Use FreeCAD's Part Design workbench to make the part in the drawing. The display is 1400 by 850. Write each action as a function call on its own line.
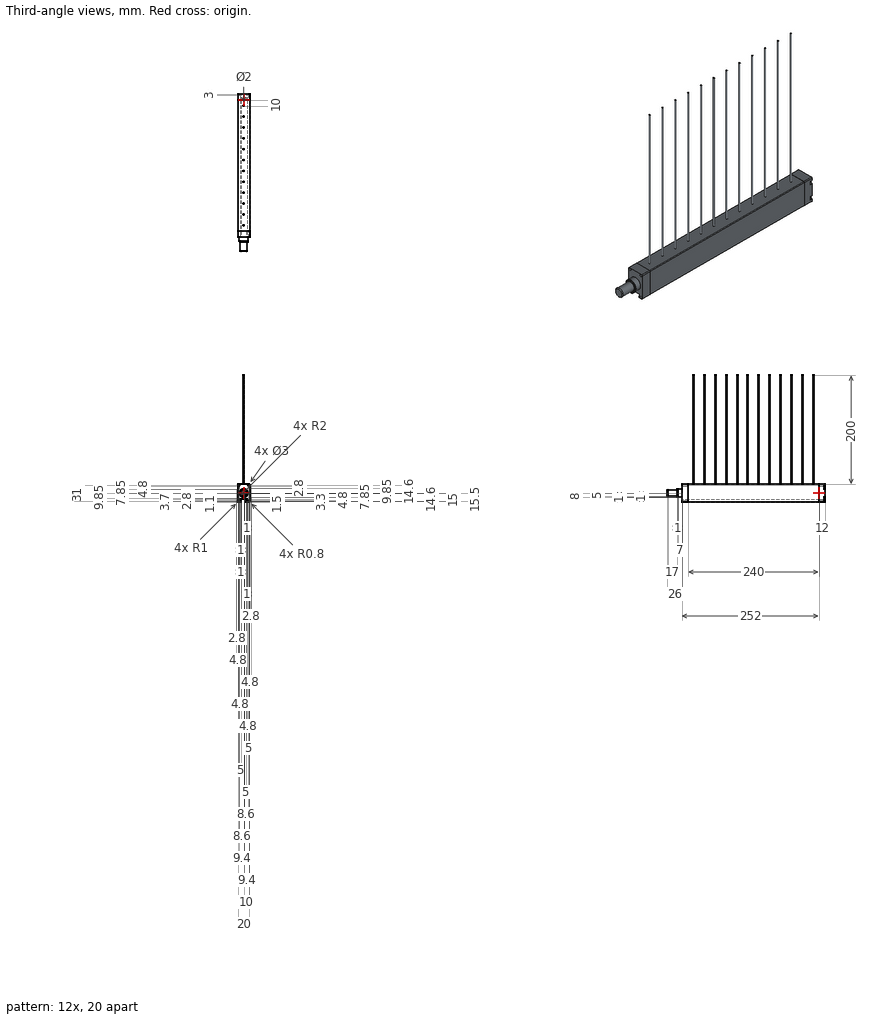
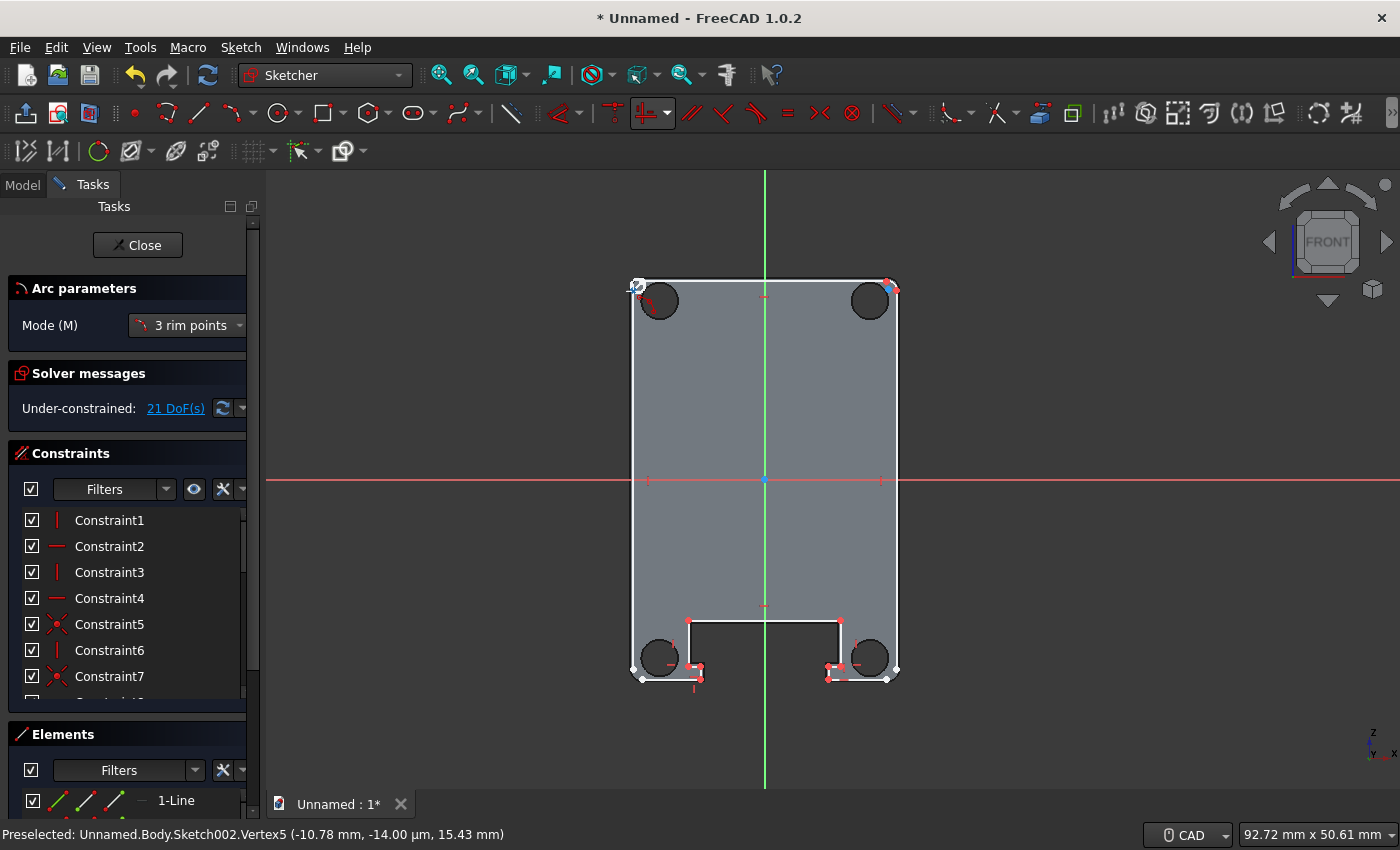
scroll(636, 283, up, 9)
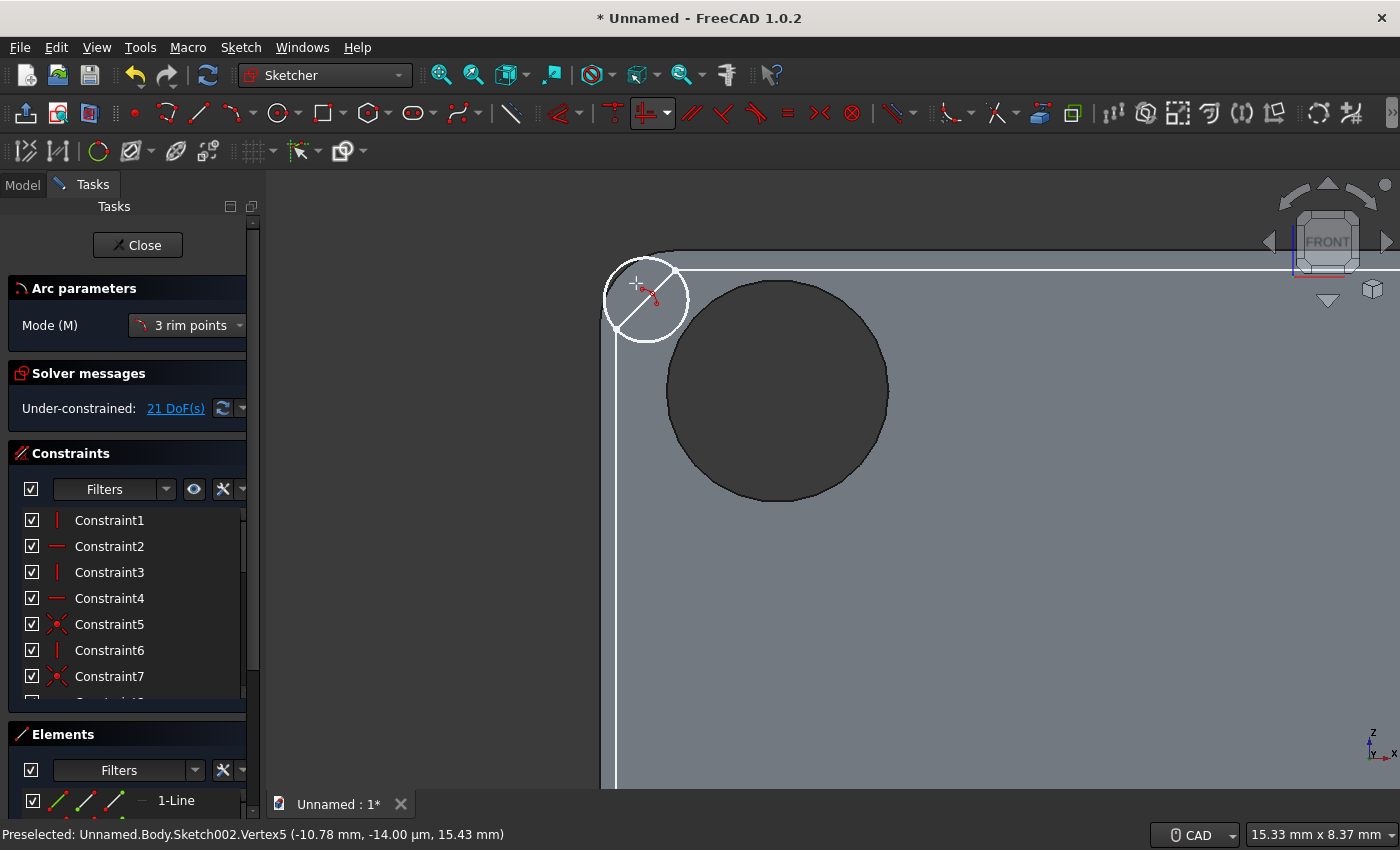
click(632, 283)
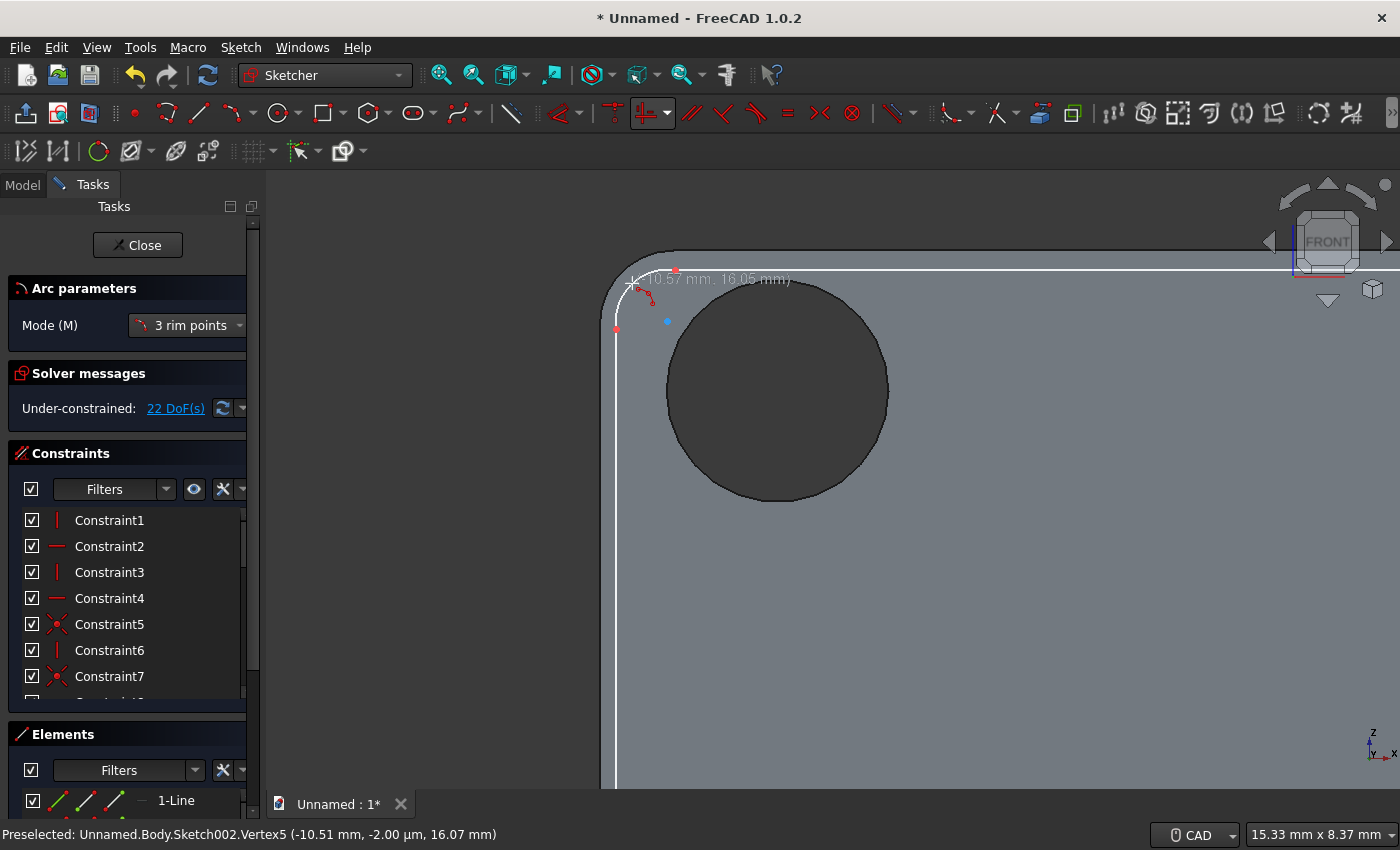
scroll(636, 283, down, 9)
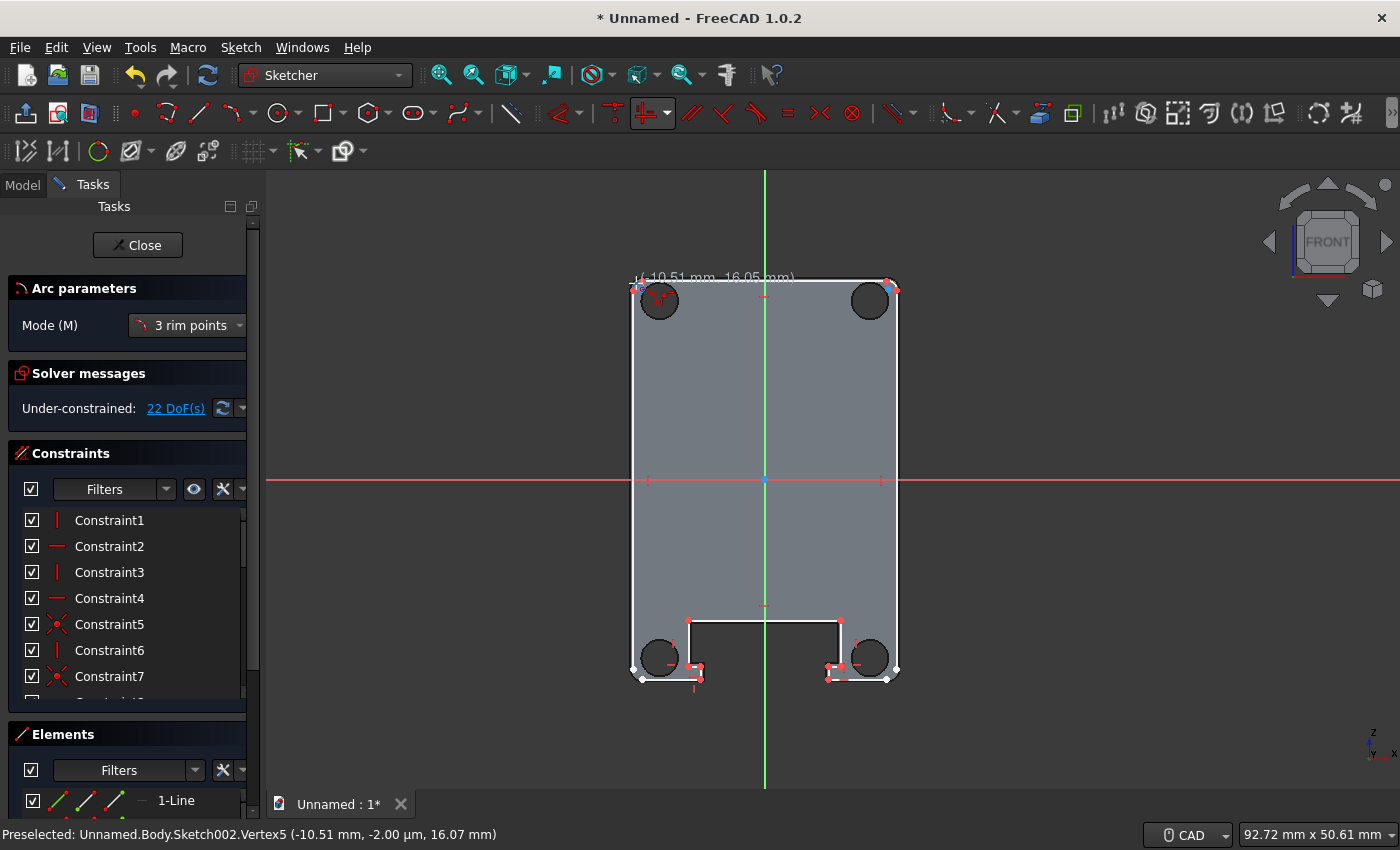
click(633, 670)
click(643, 680)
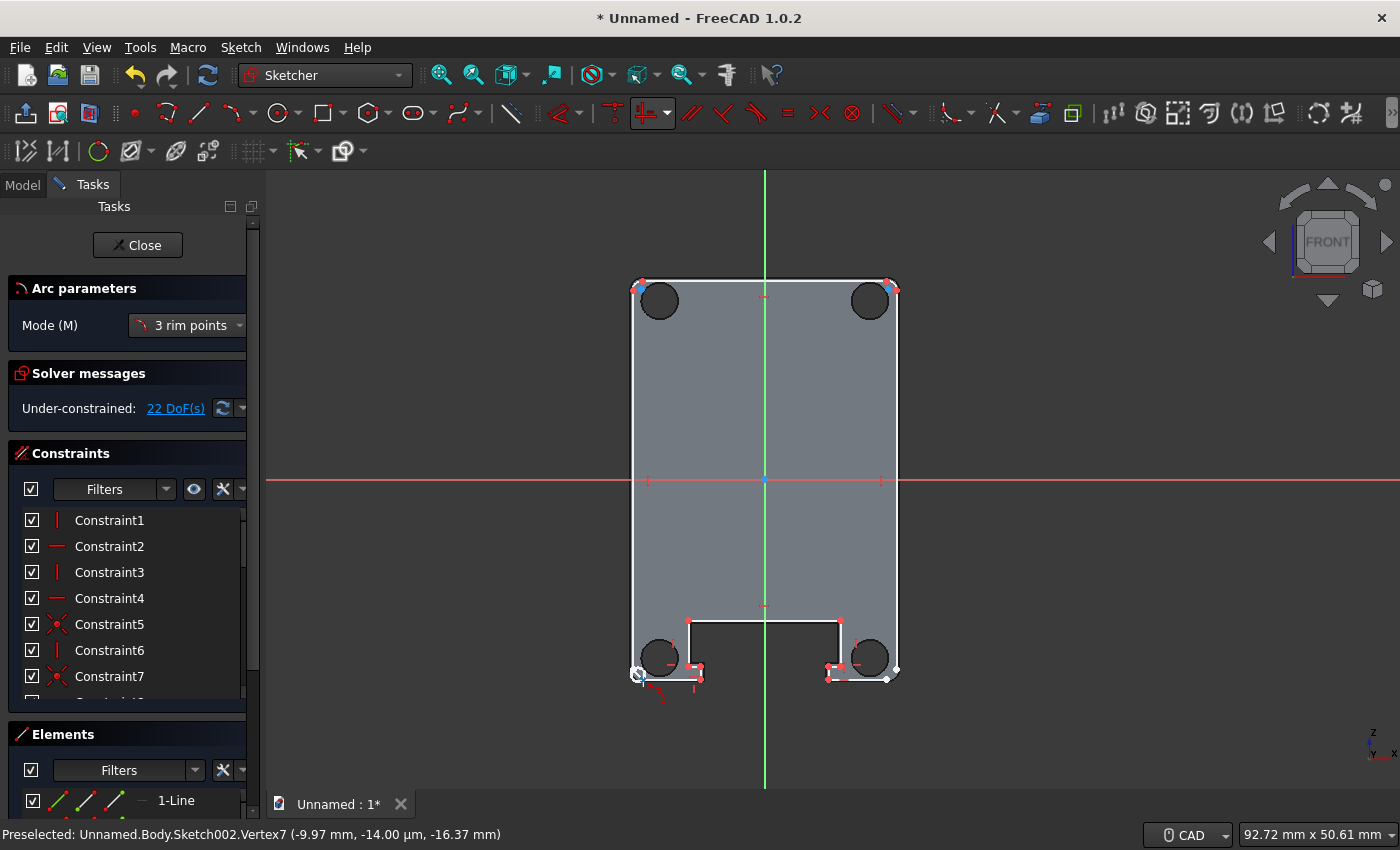
scroll(636, 676, up, 9)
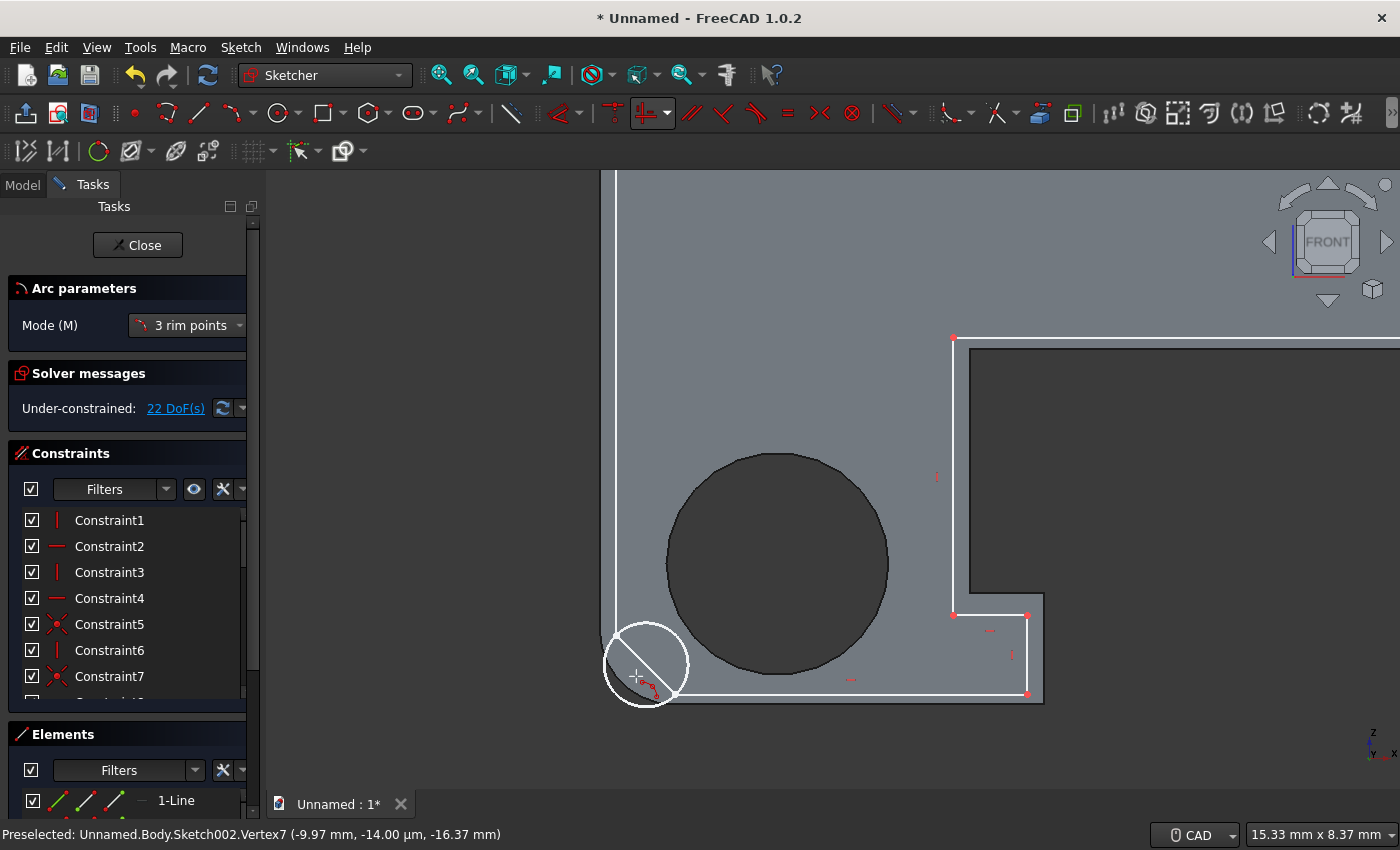
click(632, 672)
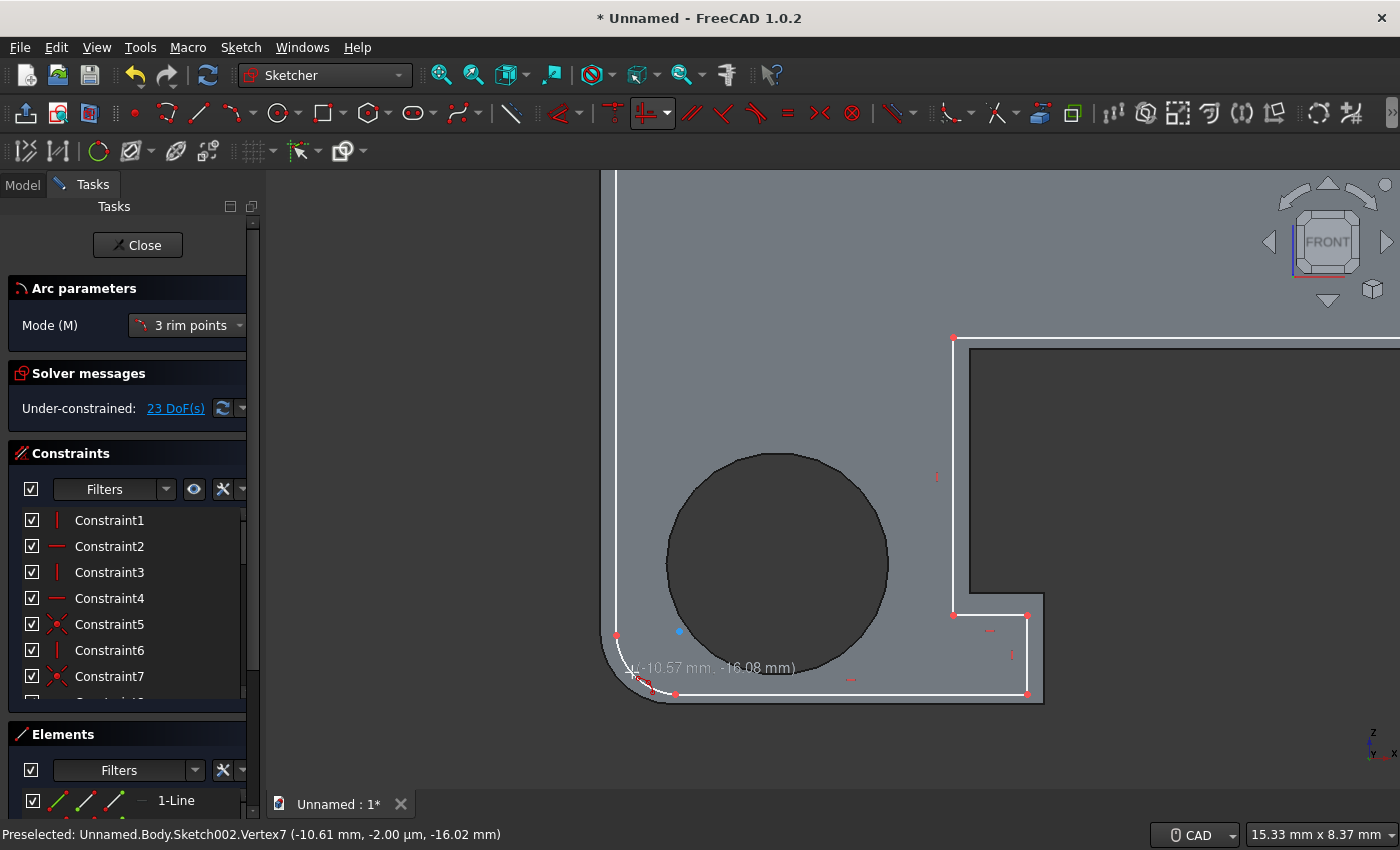
scroll(636, 677, down, 9)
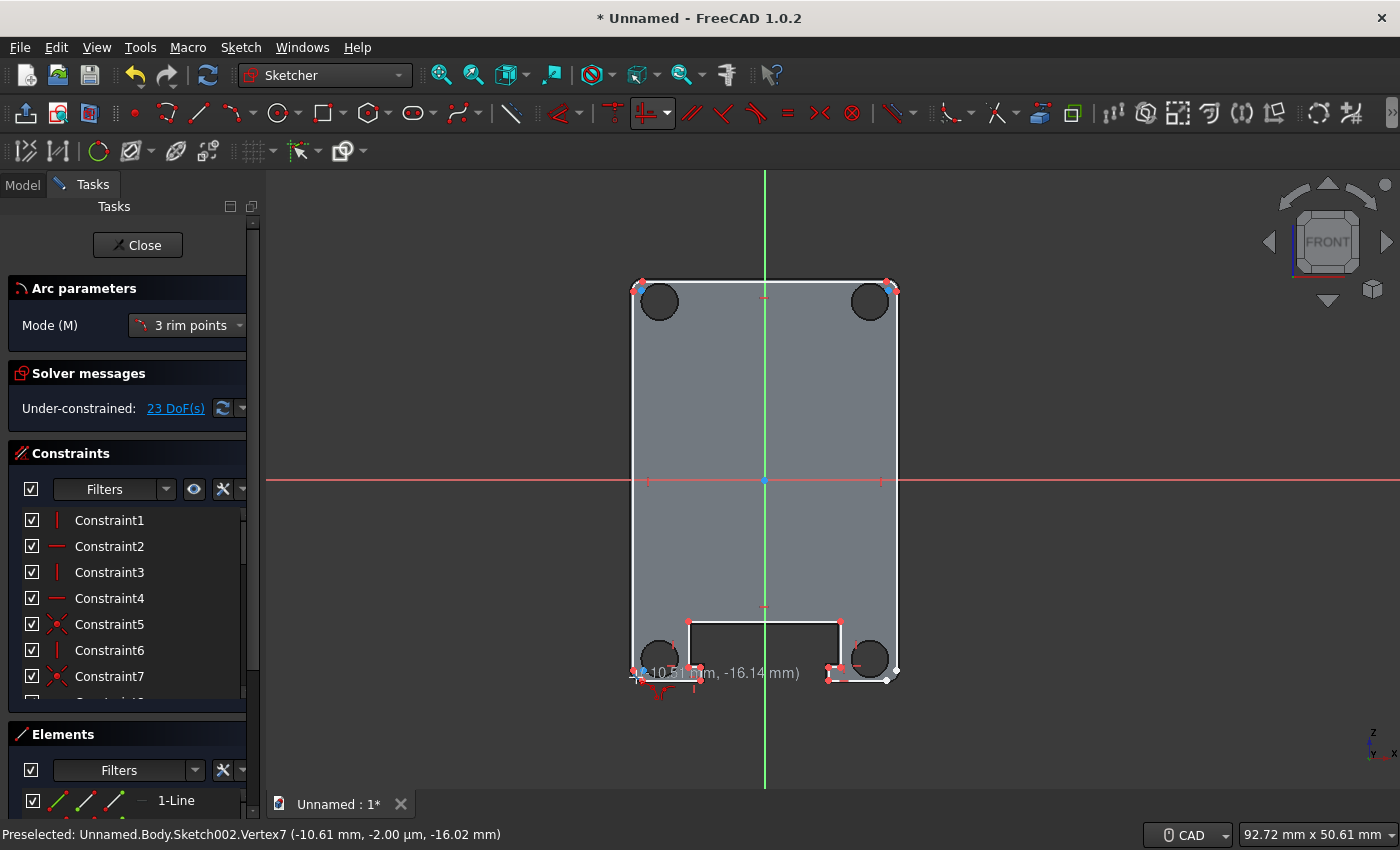
click(887, 681)
click(897, 671)